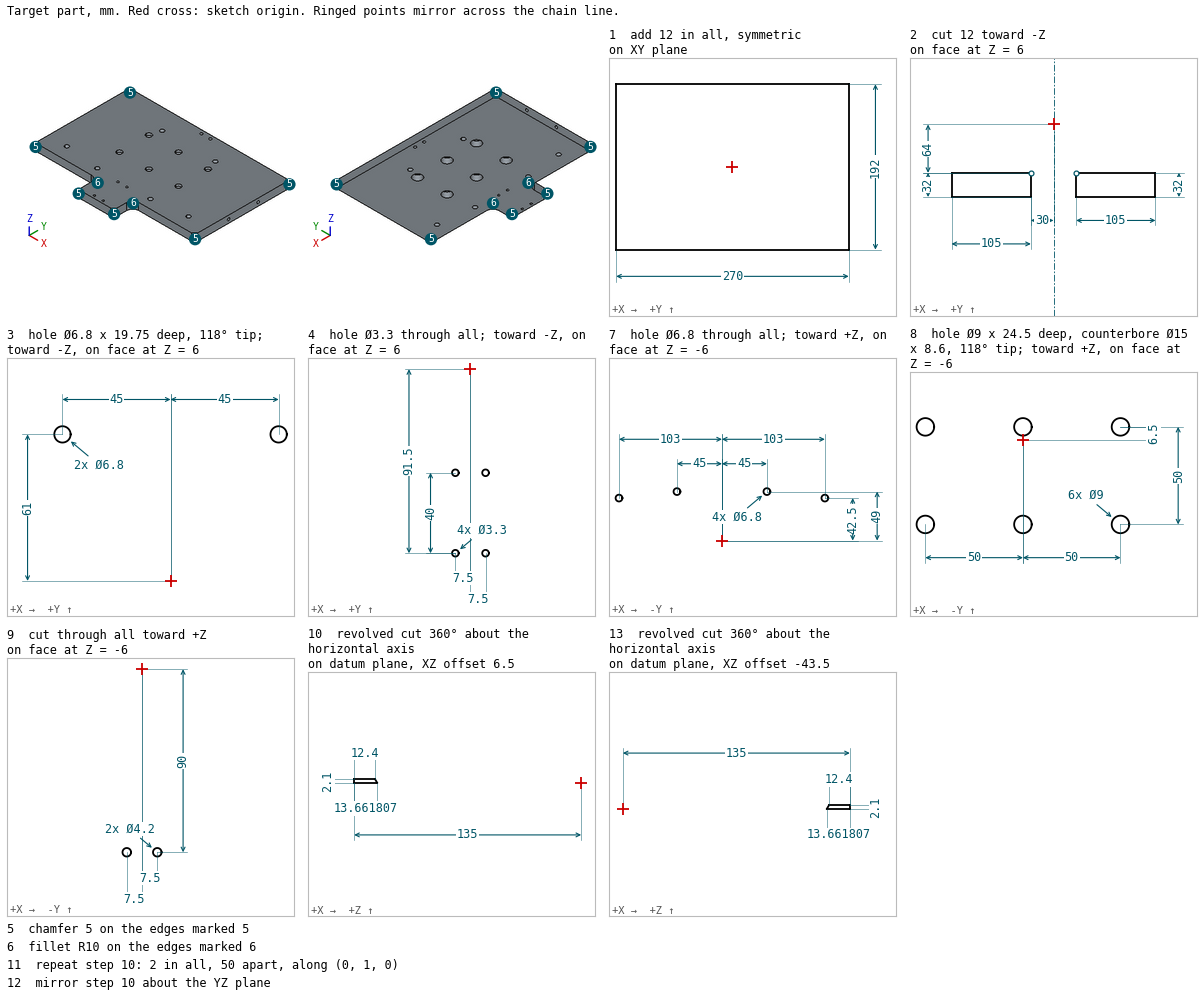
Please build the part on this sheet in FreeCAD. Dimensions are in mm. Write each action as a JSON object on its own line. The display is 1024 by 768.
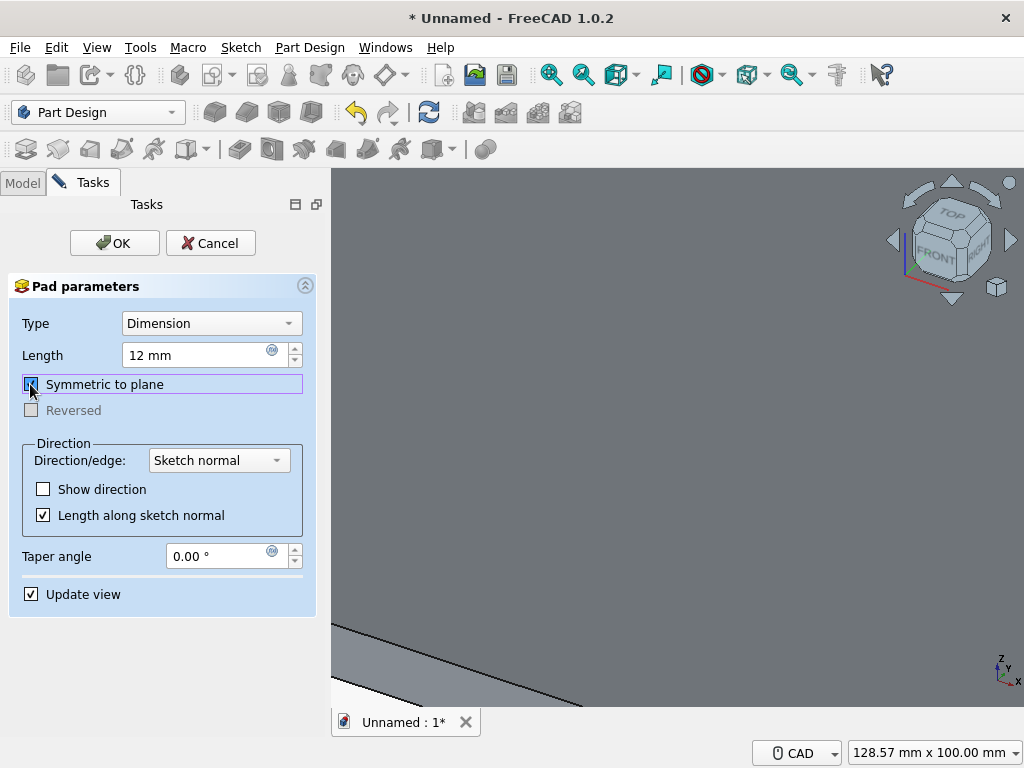
{"action": "left_click", "coordinate": [115, 243]}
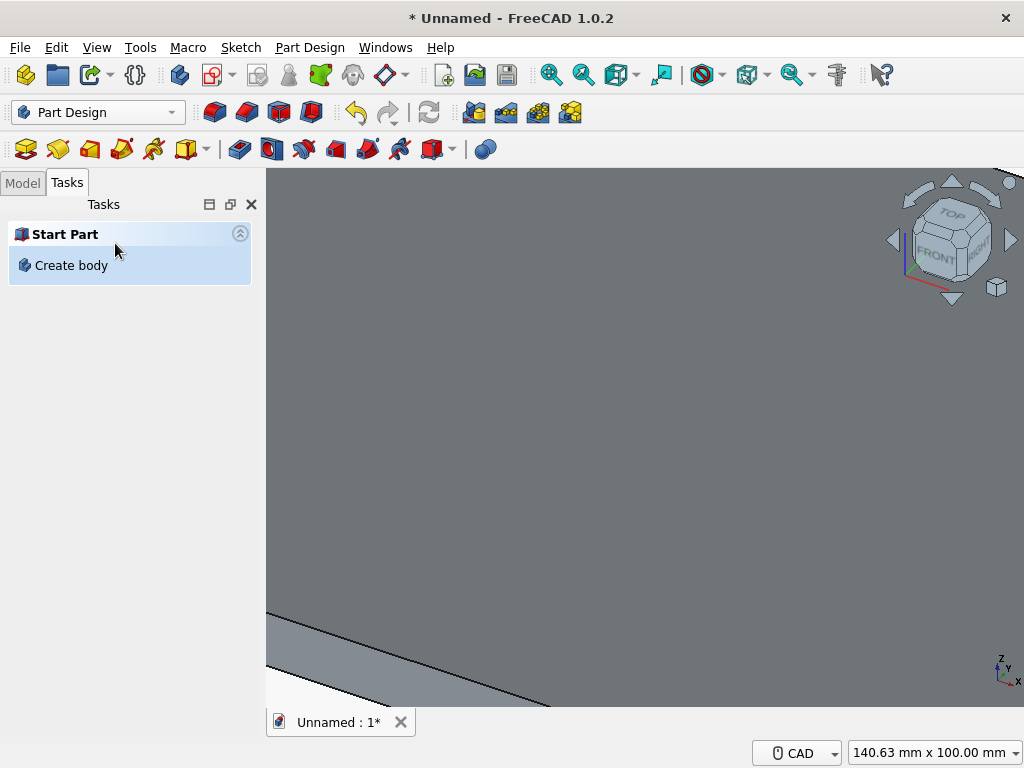
{"action": "left_click", "coordinate": [552, 76]}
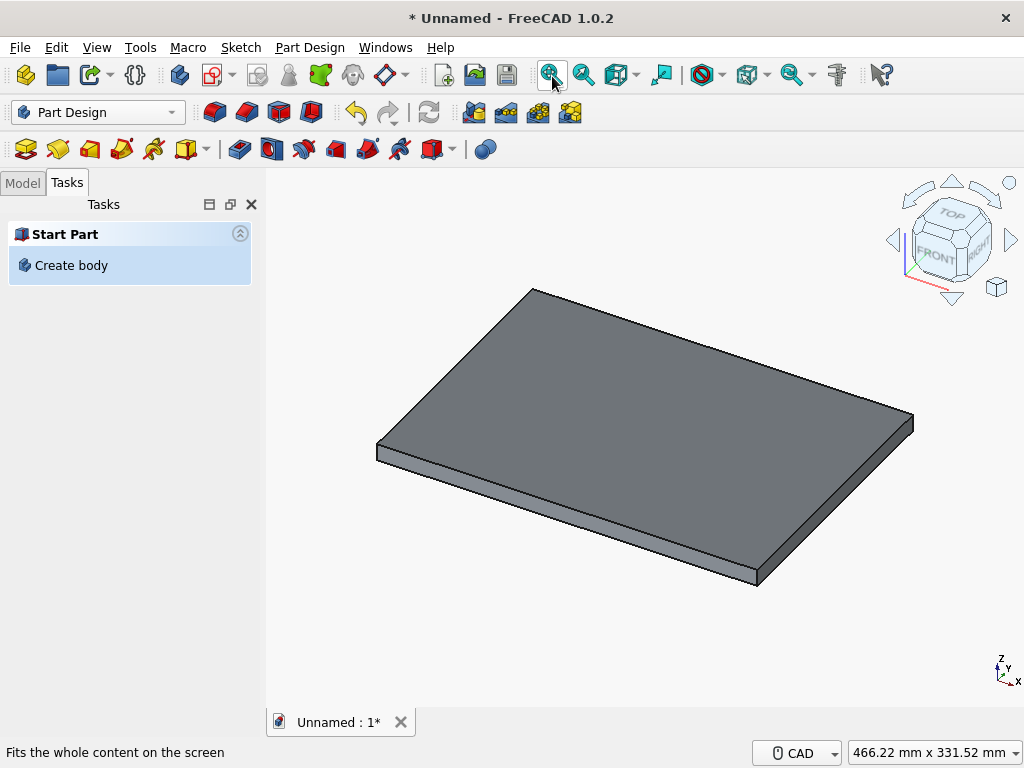
{"action": "left_click", "coordinate": [699, 446]}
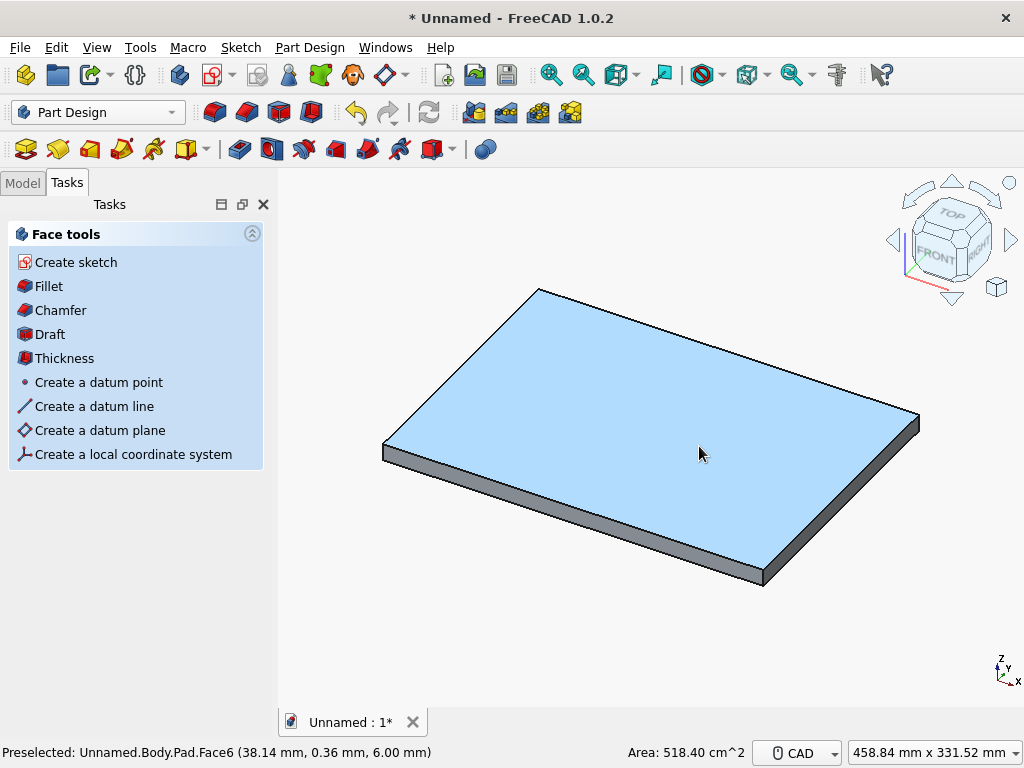
{"action": "left_click", "coordinate": [212, 76]}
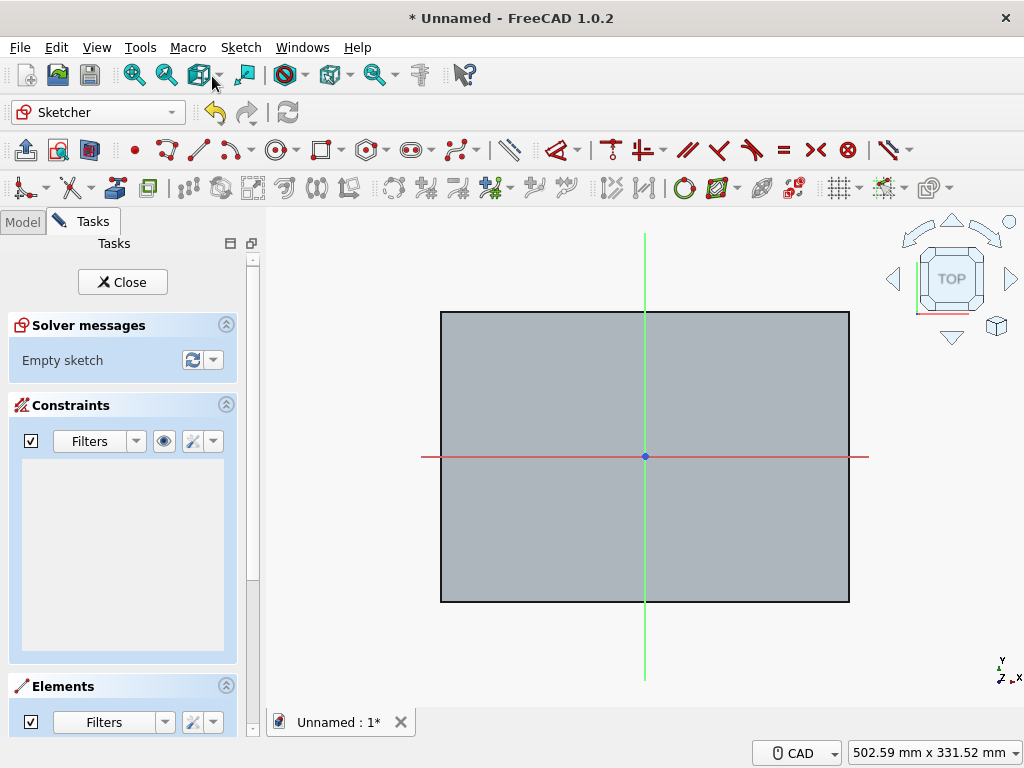
{"action": "scroll", "coordinate": [294, 235], "scroll_direction": "down", "scroll_amount": 1}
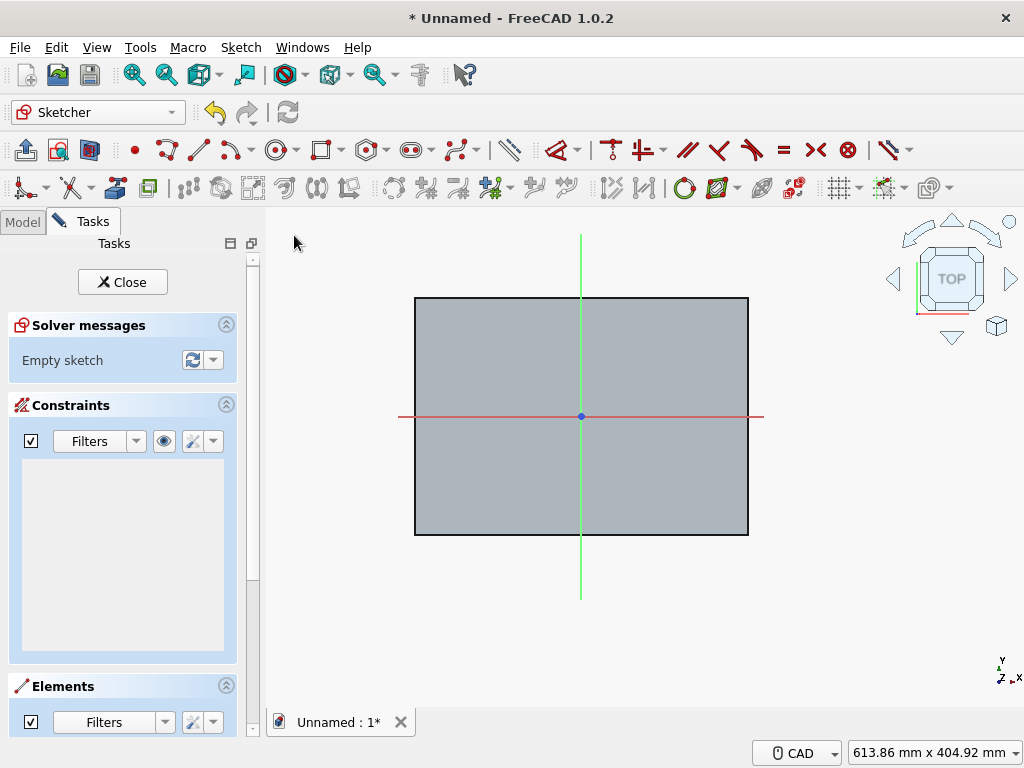
{"action": "key", "text": "g r"}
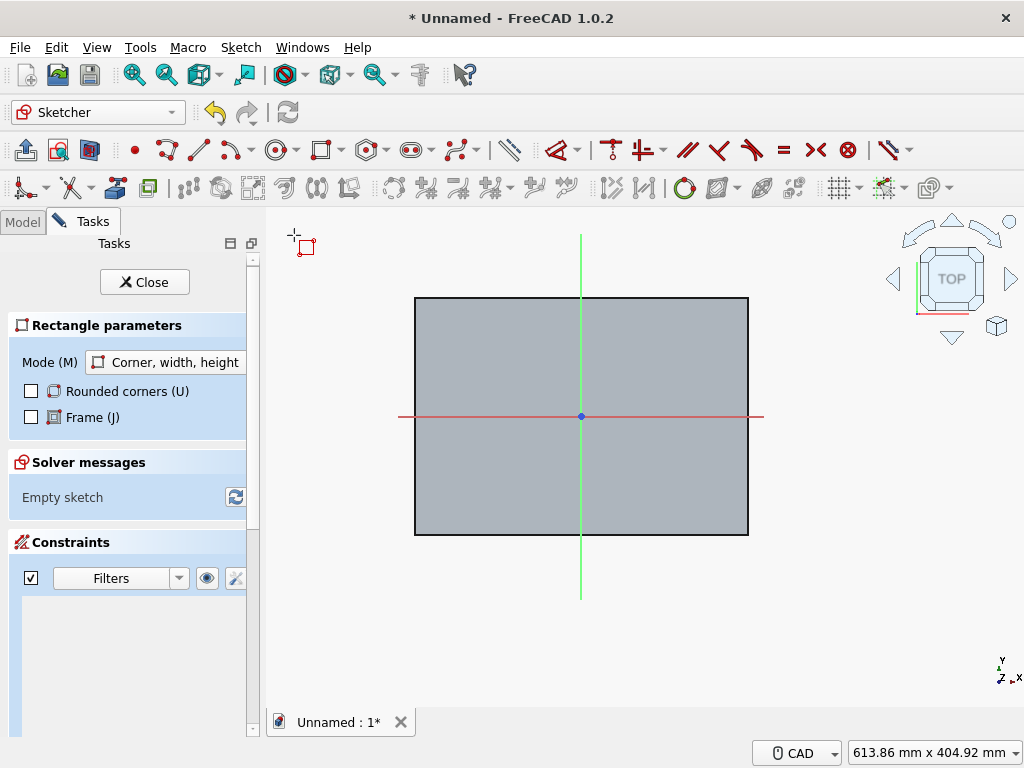
{"action": "left_click", "coordinate": [415, 496]}
{"action": "mouse_move", "coordinate": [544, 535]}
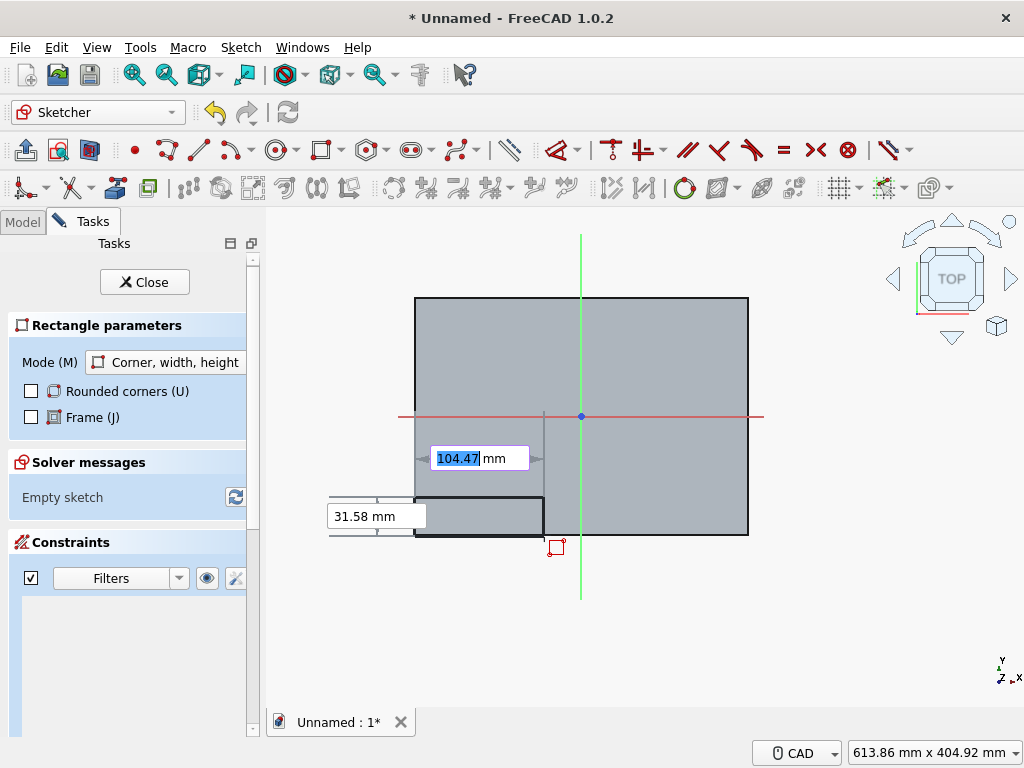
{"action": "type", "text": "105"}
{"action": "key", "text": "Tab"}
{"action": "type", "text": "32"}
{"action": "key", "text": "Return"}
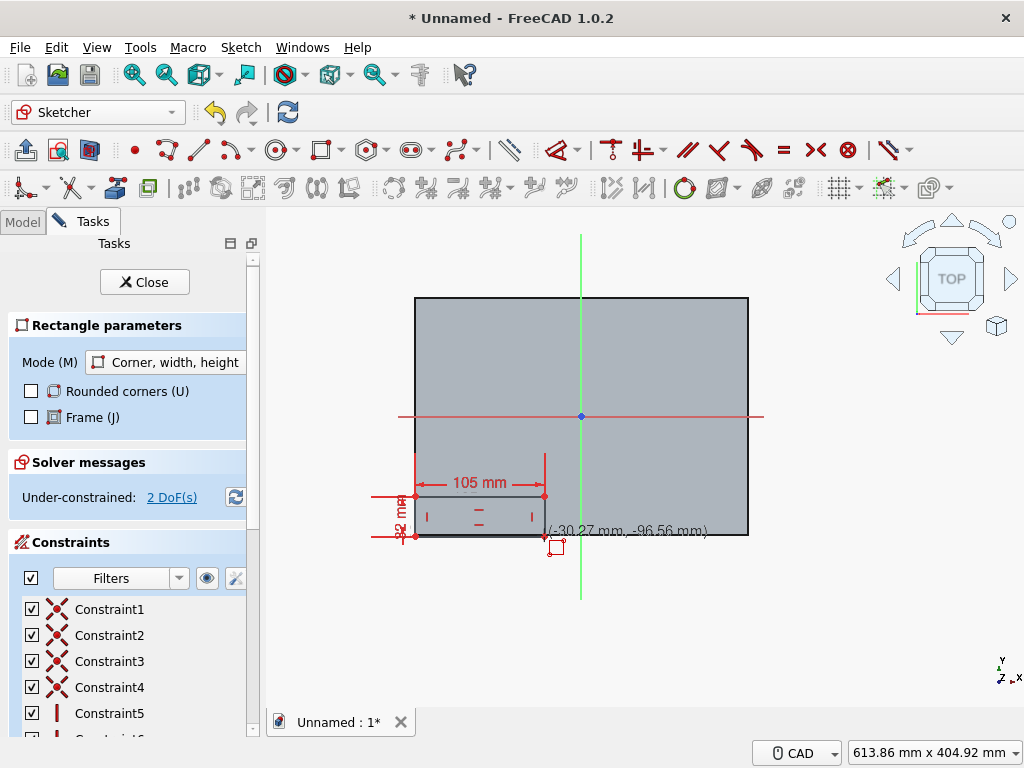
{"action": "left_click", "coordinate": [618, 496]}
{"action": "mouse_move", "coordinate": [748, 535]}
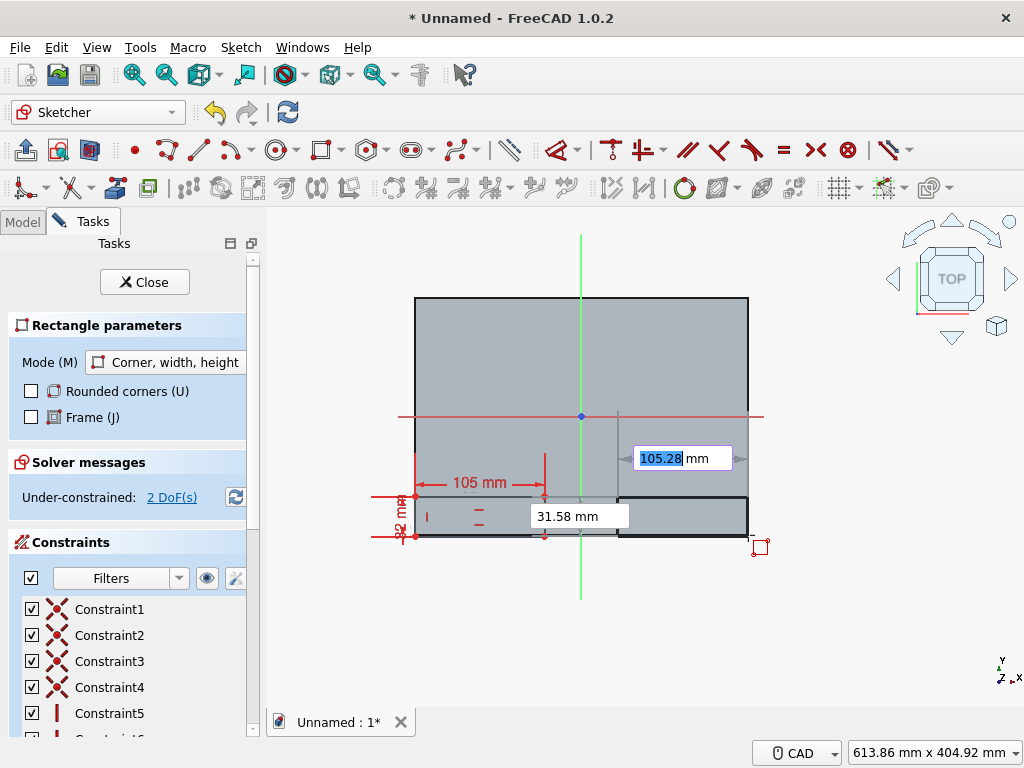
{"action": "type", "text": "105"}
{"action": "key", "text": "Tab"}
{"action": "type", "text": "32"}
{"action": "key", "text": "Return"}
{"action": "key", "text": "Escape"}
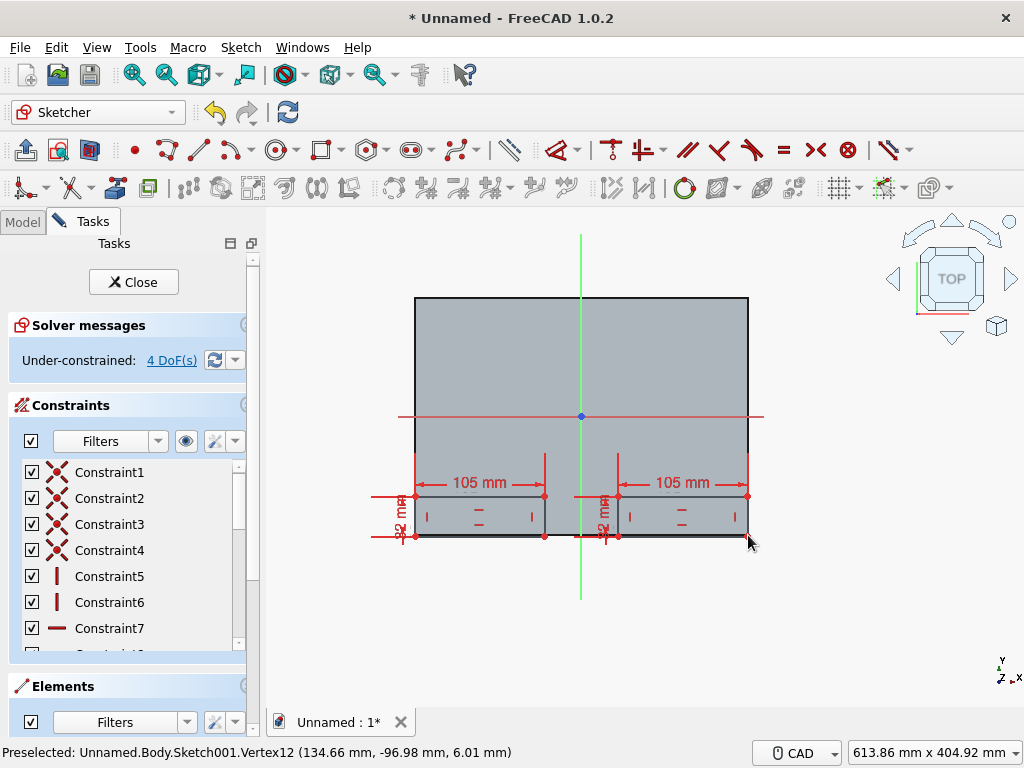
{"action": "left_click", "coordinate": [545, 497]}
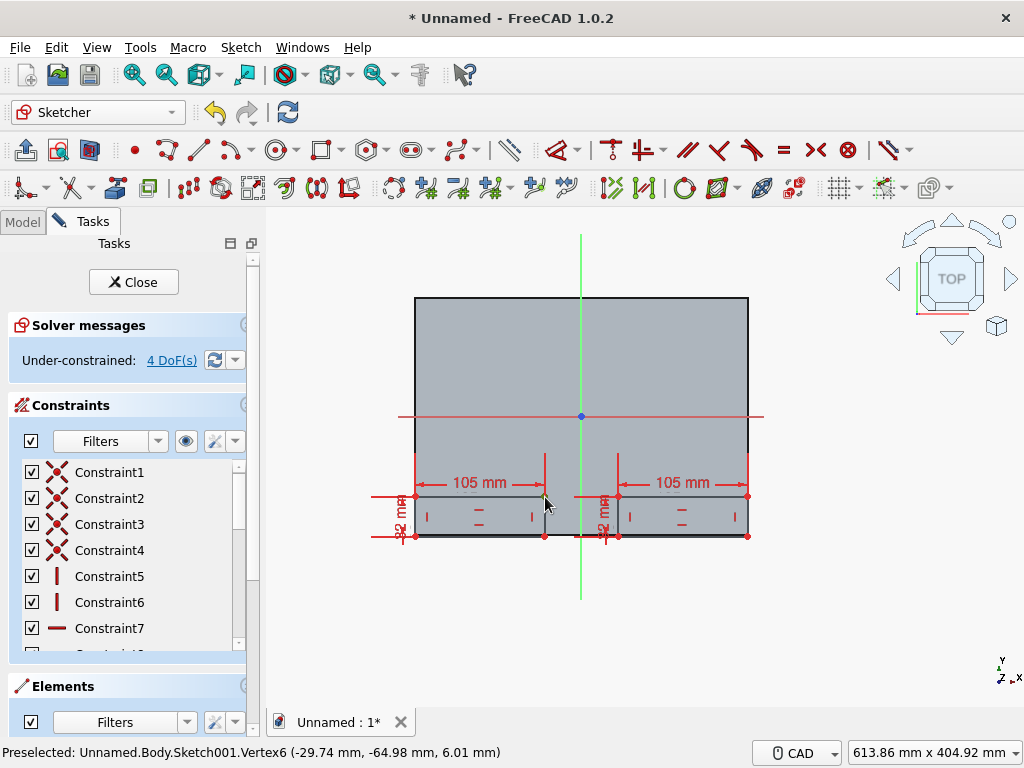
{"action": "left_click", "coordinate": [618, 497]}